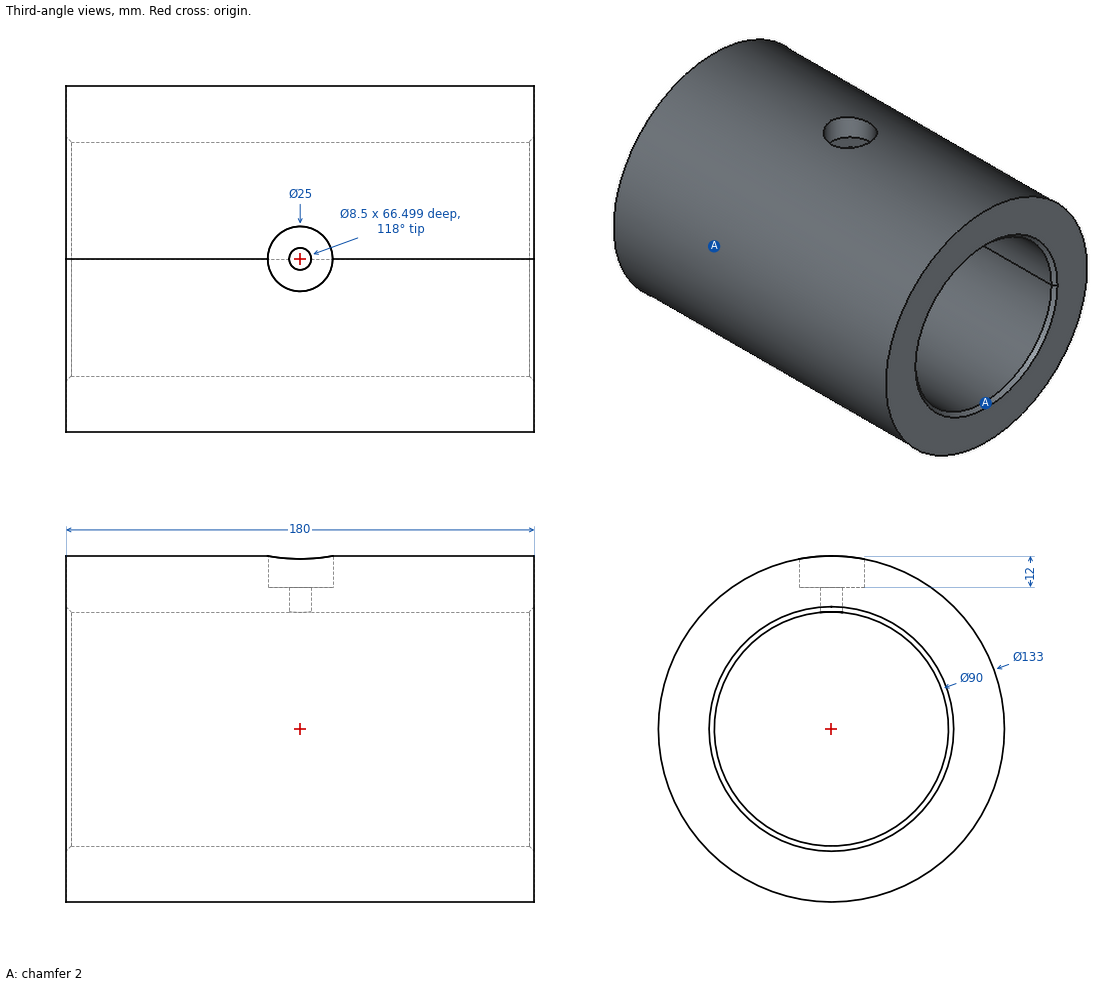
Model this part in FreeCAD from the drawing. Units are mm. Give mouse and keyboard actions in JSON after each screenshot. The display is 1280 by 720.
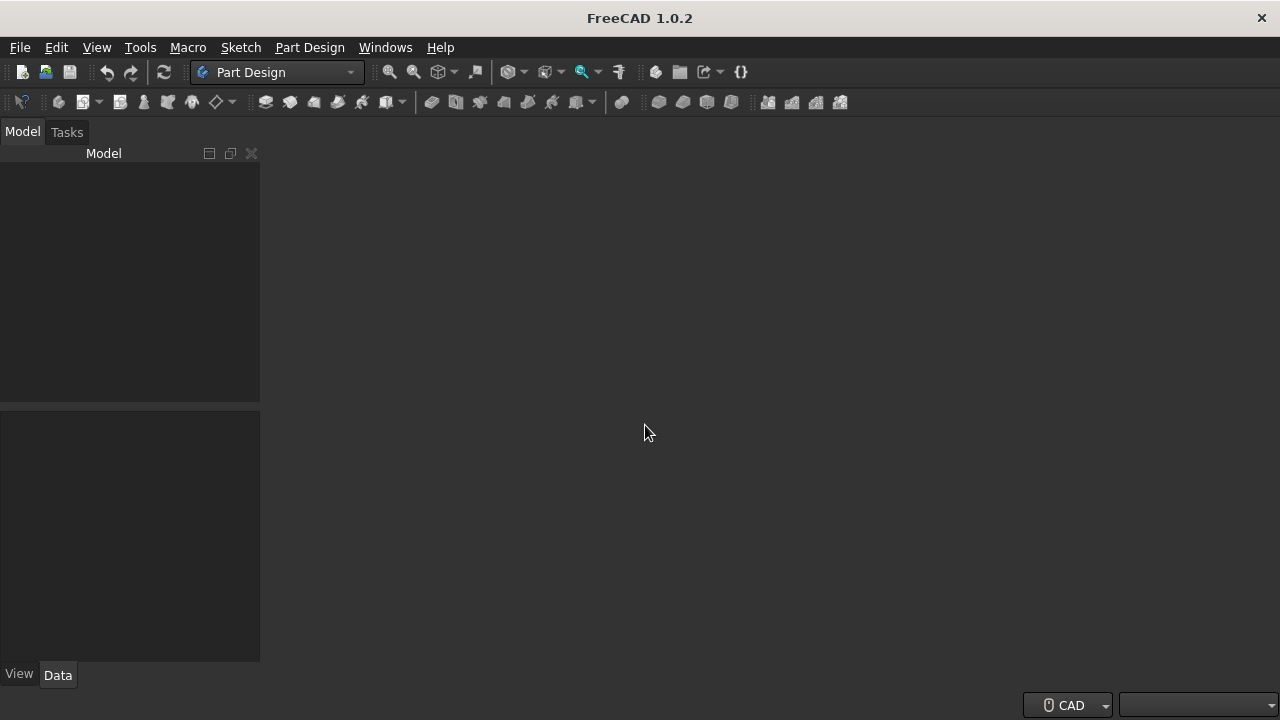
{"action": "left_click", "coordinate": [22, 72]}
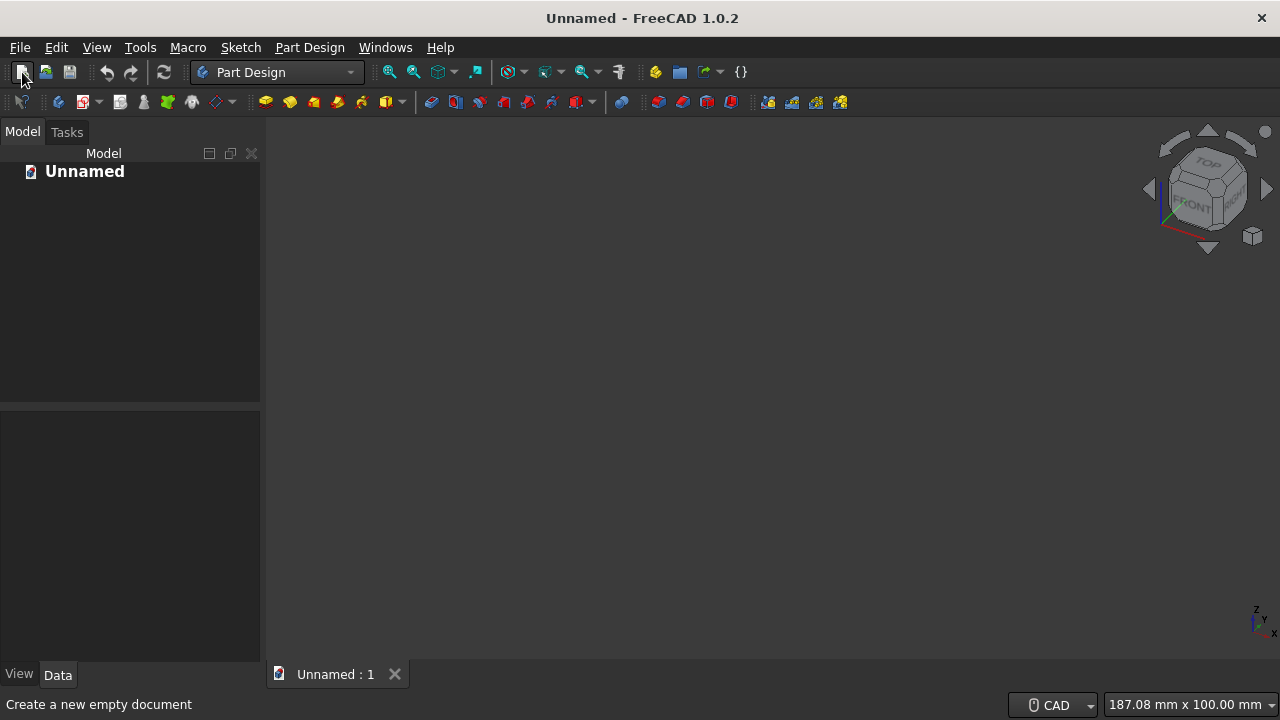
{"action": "left_click", "coordinate": [84, 102]}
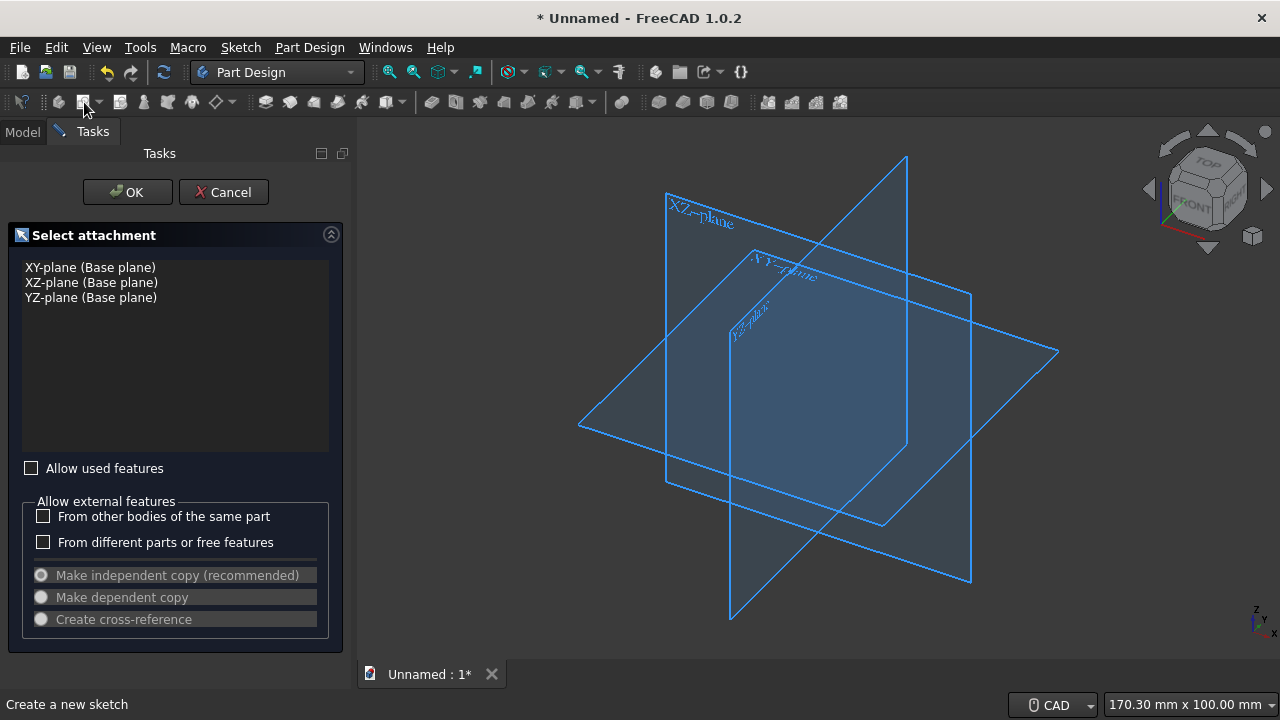
{"action": "left_click", "coordinate": [82, 298]}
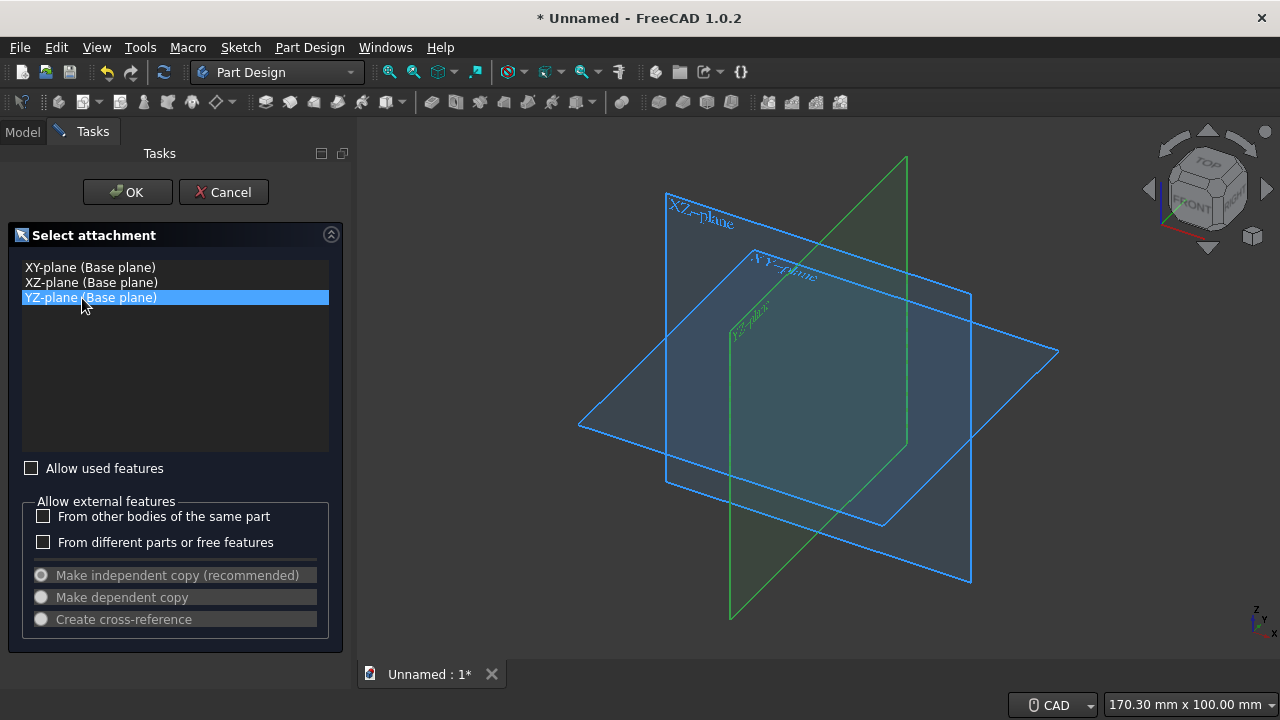
{"action": "left_click", "coordinate": [128, 192]}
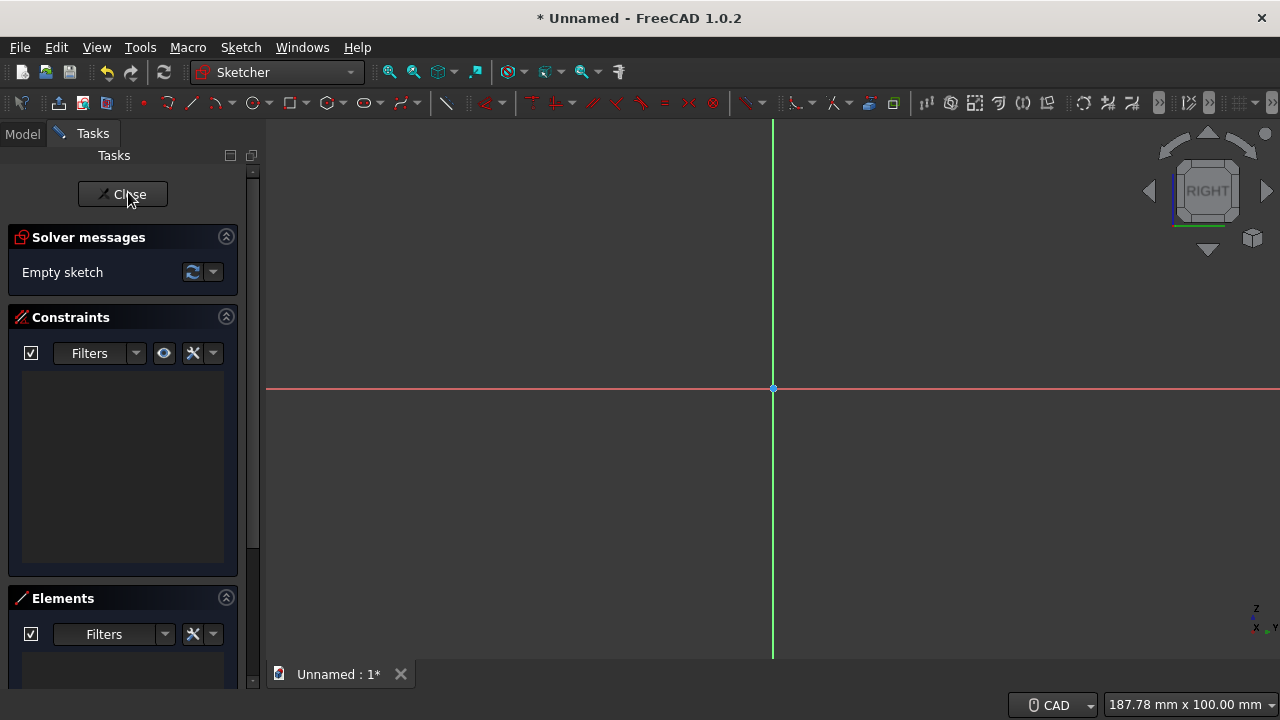
{"action": "scroll", "coordinate": [649, 389], "scroll_direction": "down", "scroll_amount": 4}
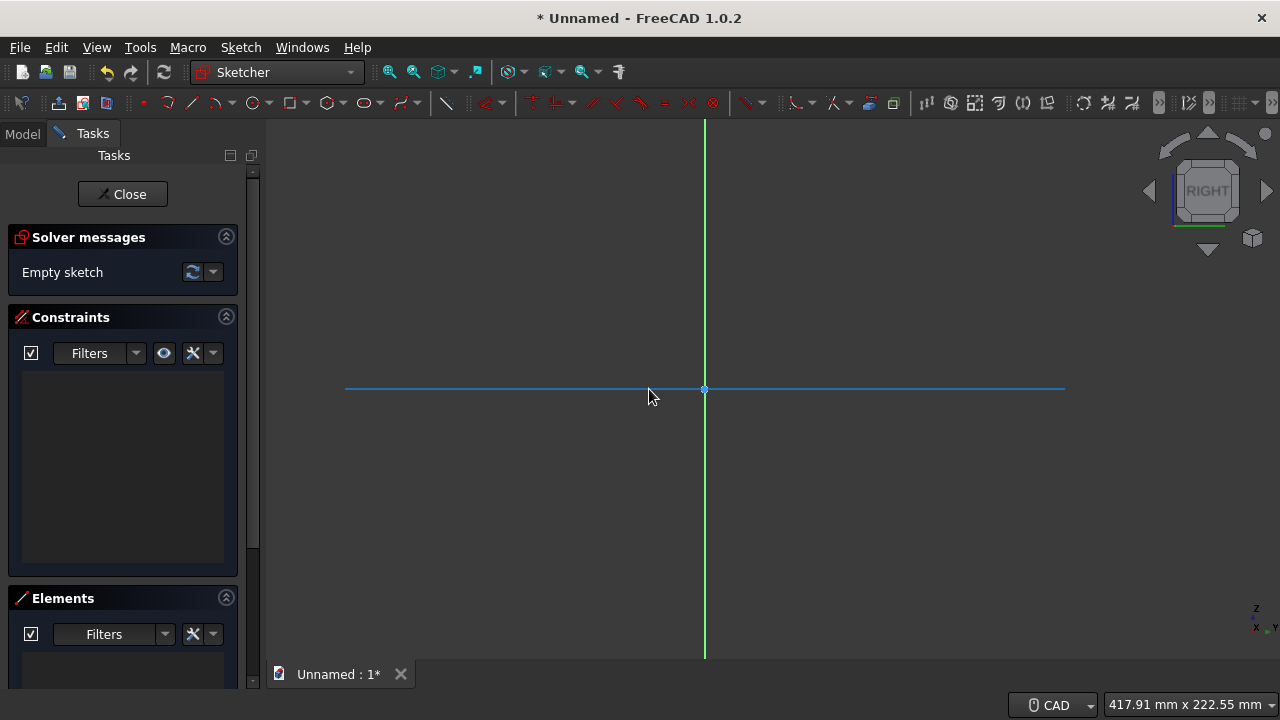
{"action": "left_click", "coordinate": [254, 104]}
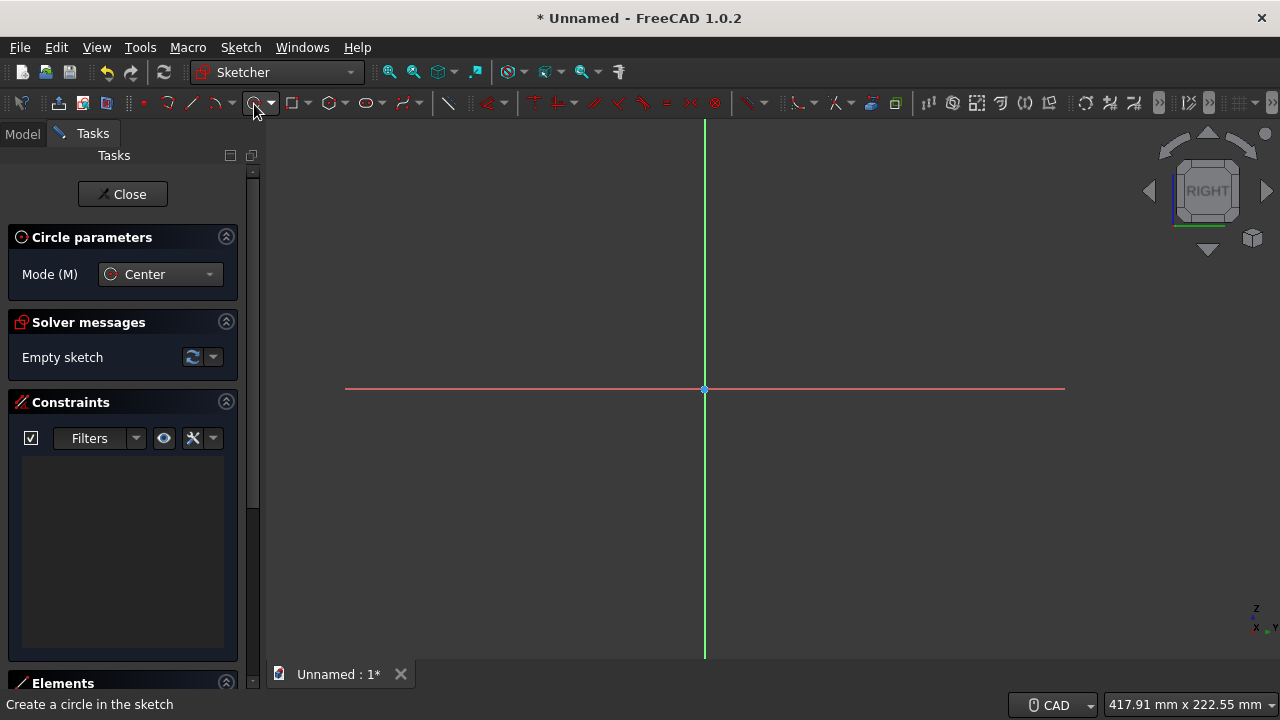
{"action": "left_click", "coordinate": [705, 389]}
{"action": "mouse_move", "coordinate": [819, 275]}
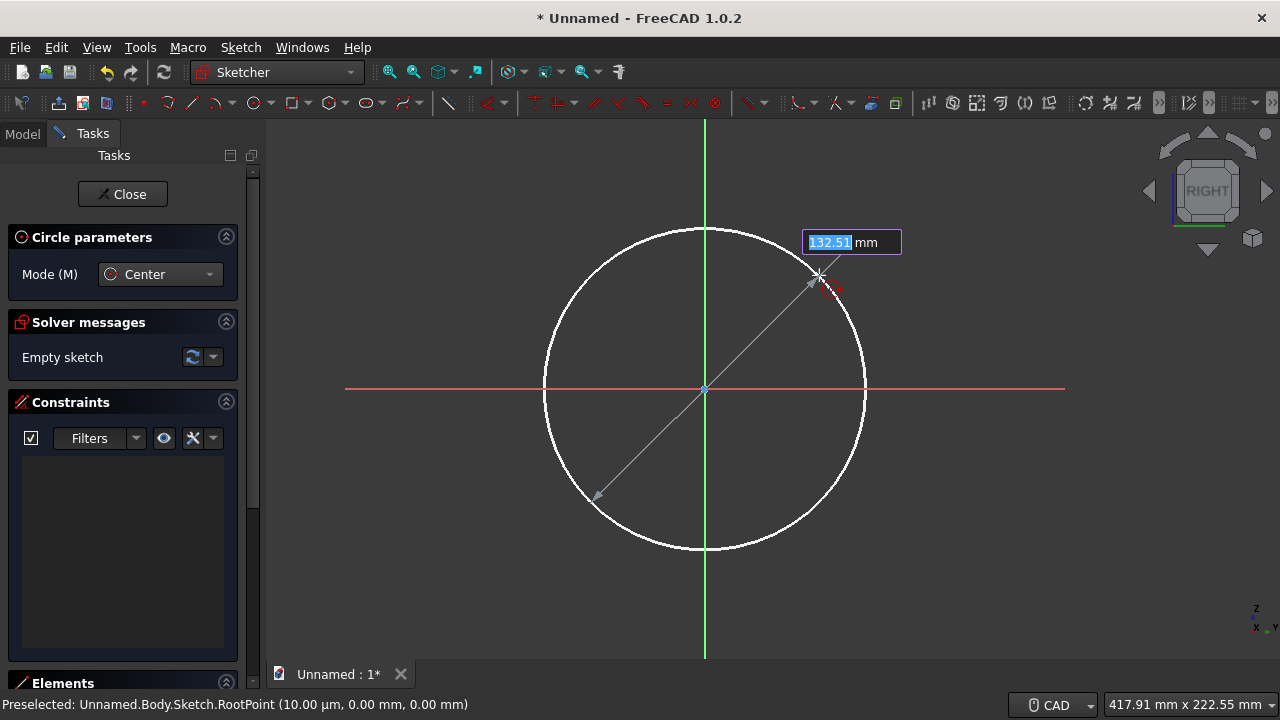
{"action": "type", "text": "133"}
{"action": "key", "text": "Return"}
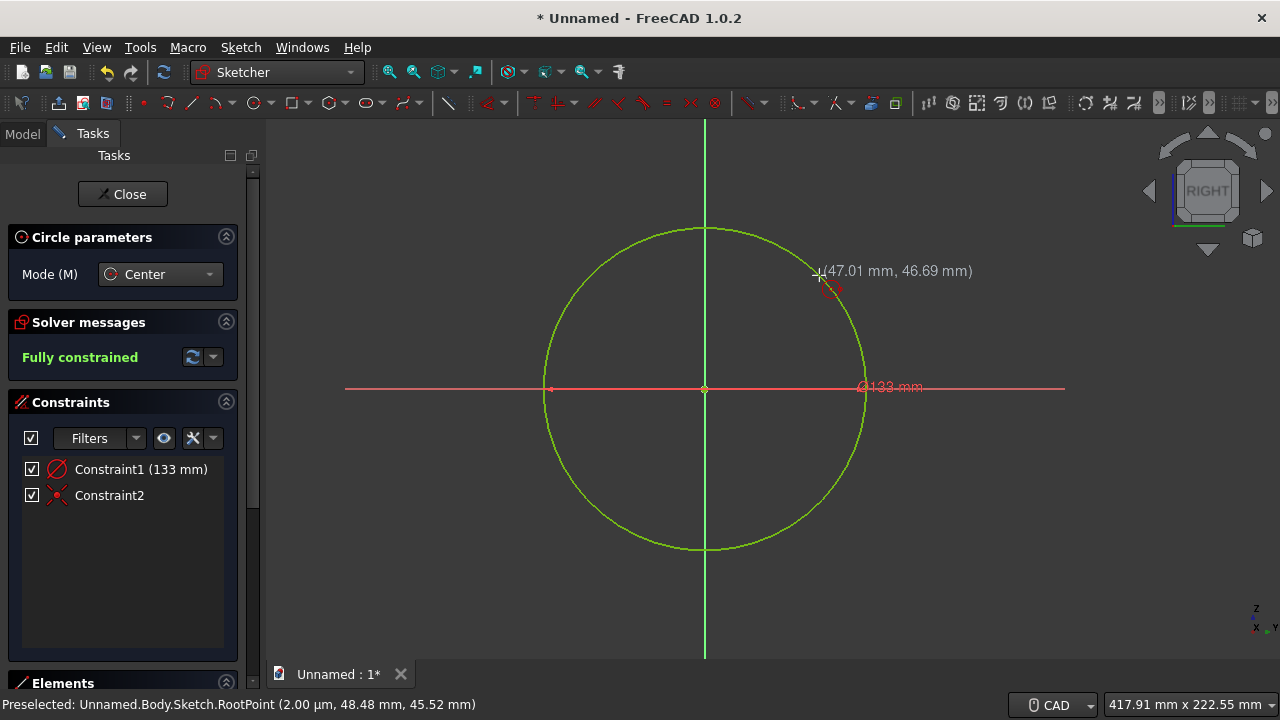
{"action": "left_click", "coordinate": [705, 389]}
{"action": "mouse_move", "coordinate": [782, 312]}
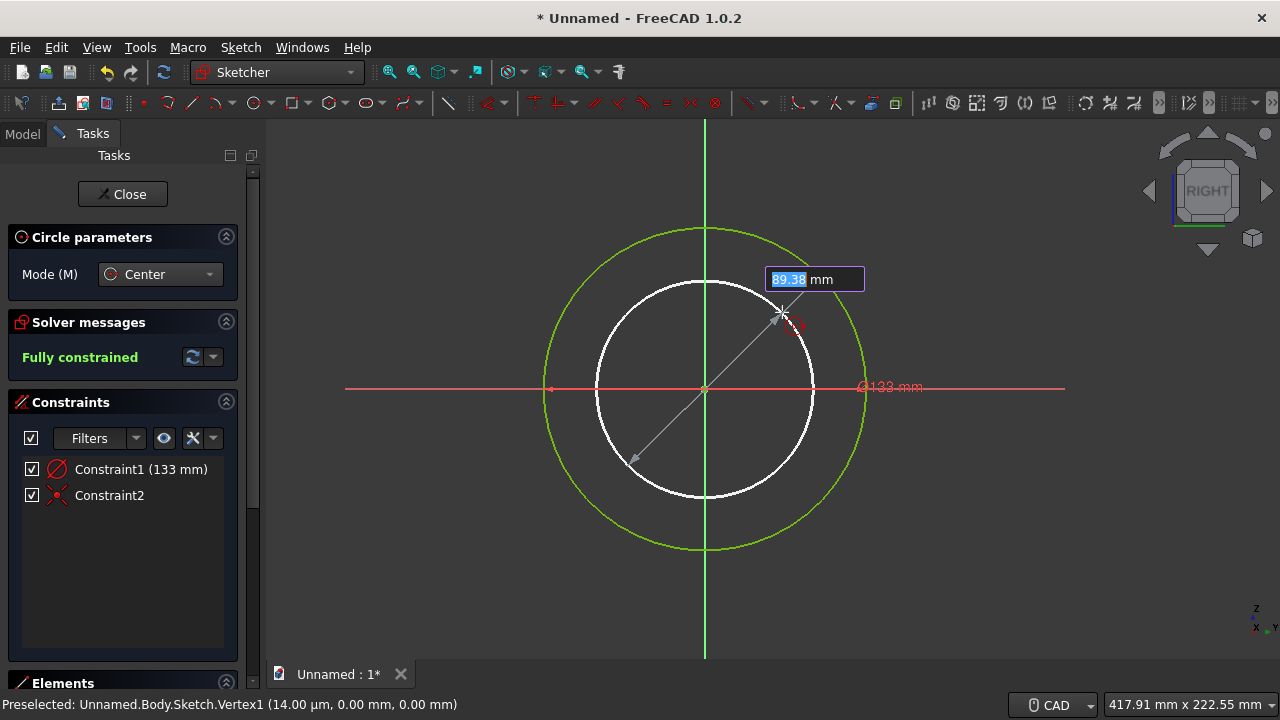
{"action": "type", "text": "90"}
{"action": "key", "text": "Return"}
{"action": "key", "text": "Escape"}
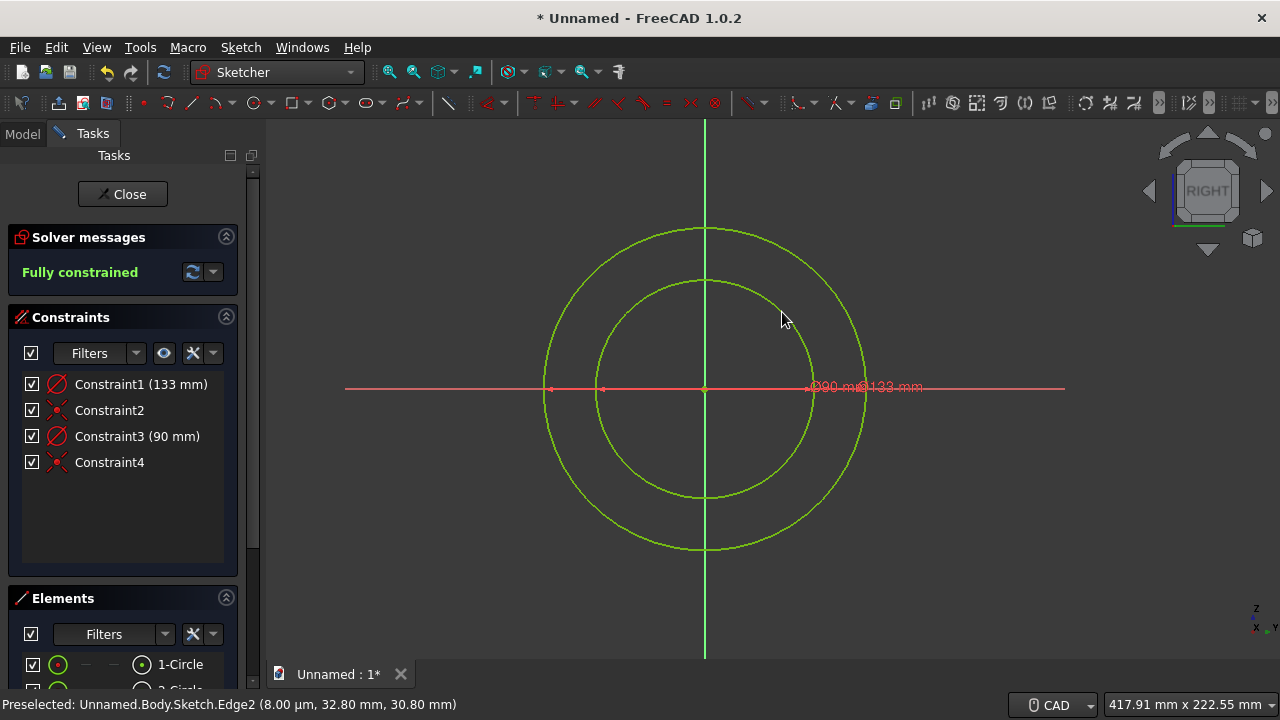
{"action": "left_click", "coordinate": [123, 194]}